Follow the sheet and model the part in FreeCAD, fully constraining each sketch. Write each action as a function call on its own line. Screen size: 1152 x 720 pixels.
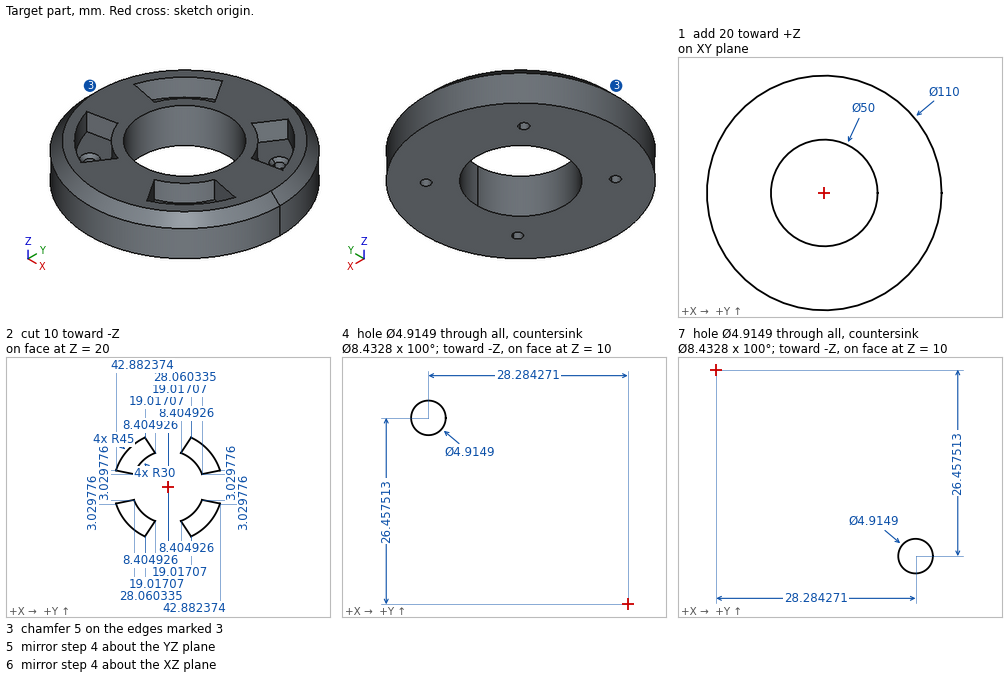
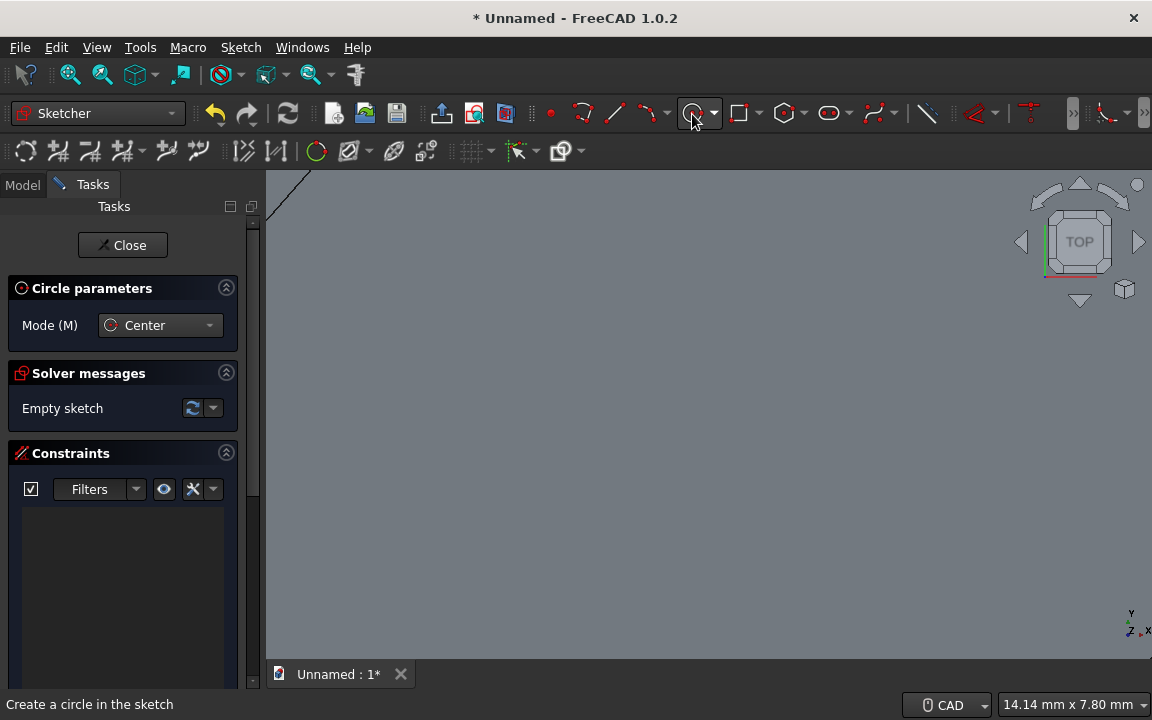
click(625, 402)
click(734, 293)
key(Escape)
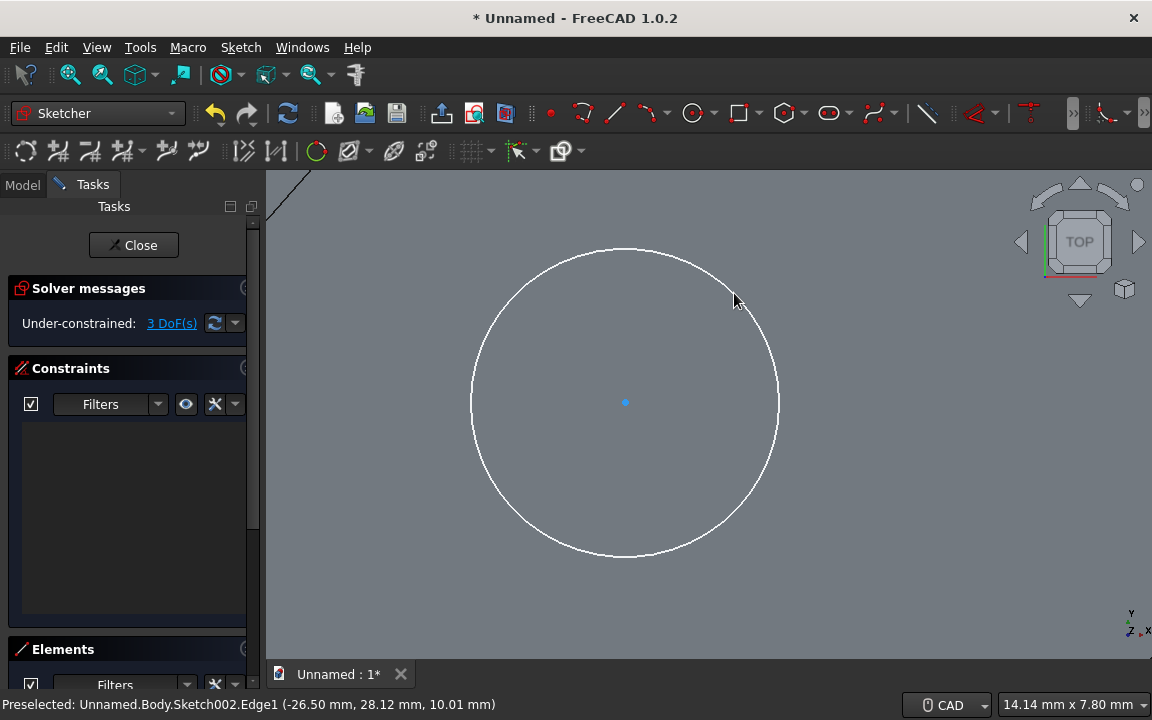
click(974, 114)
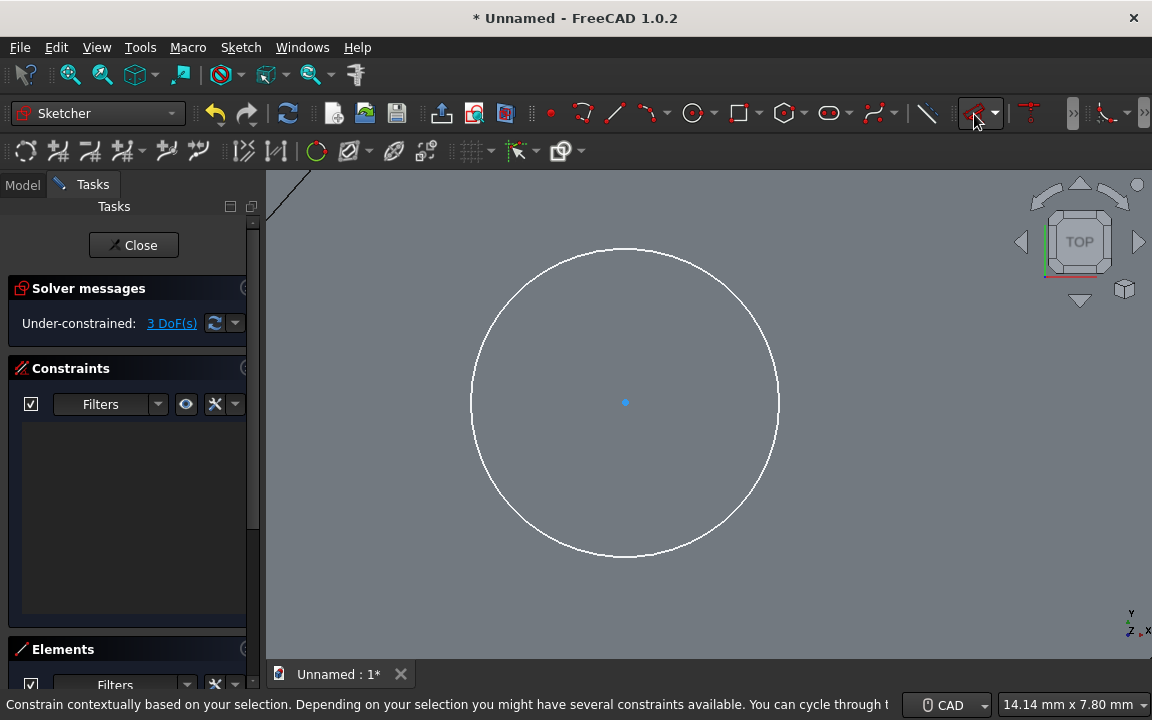
click(734, 294)
click(757, 271)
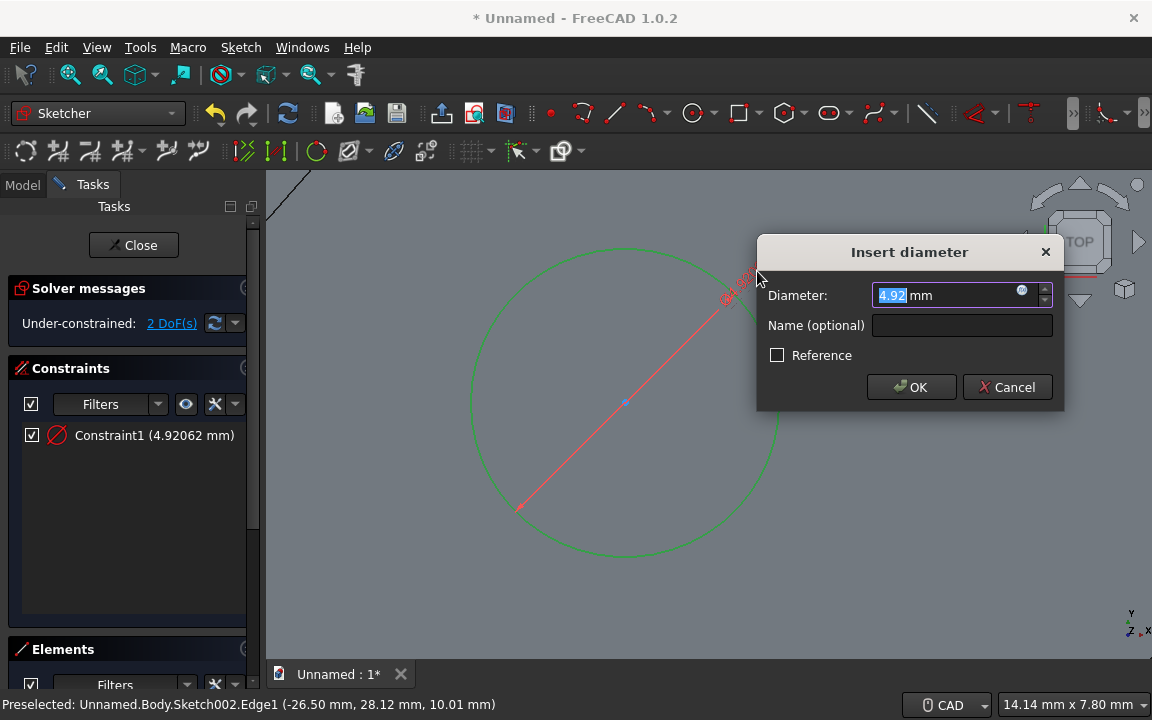
text(4.9149)
key(Return)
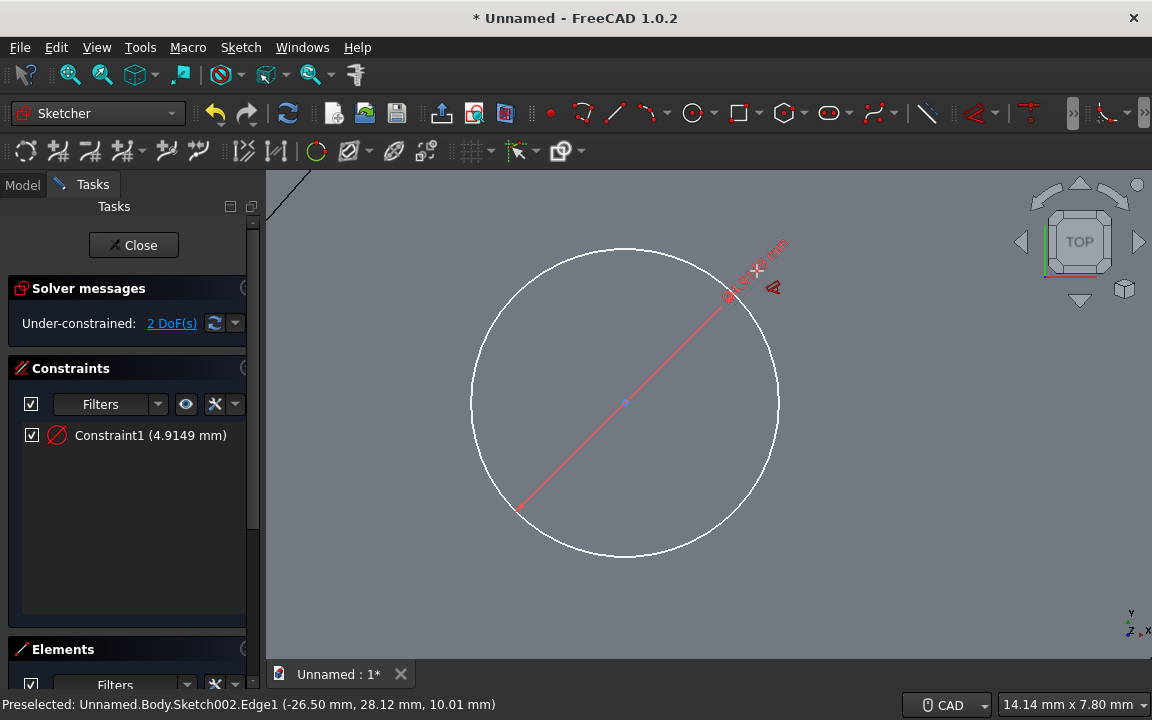
click(625, 403)
click(806, 369)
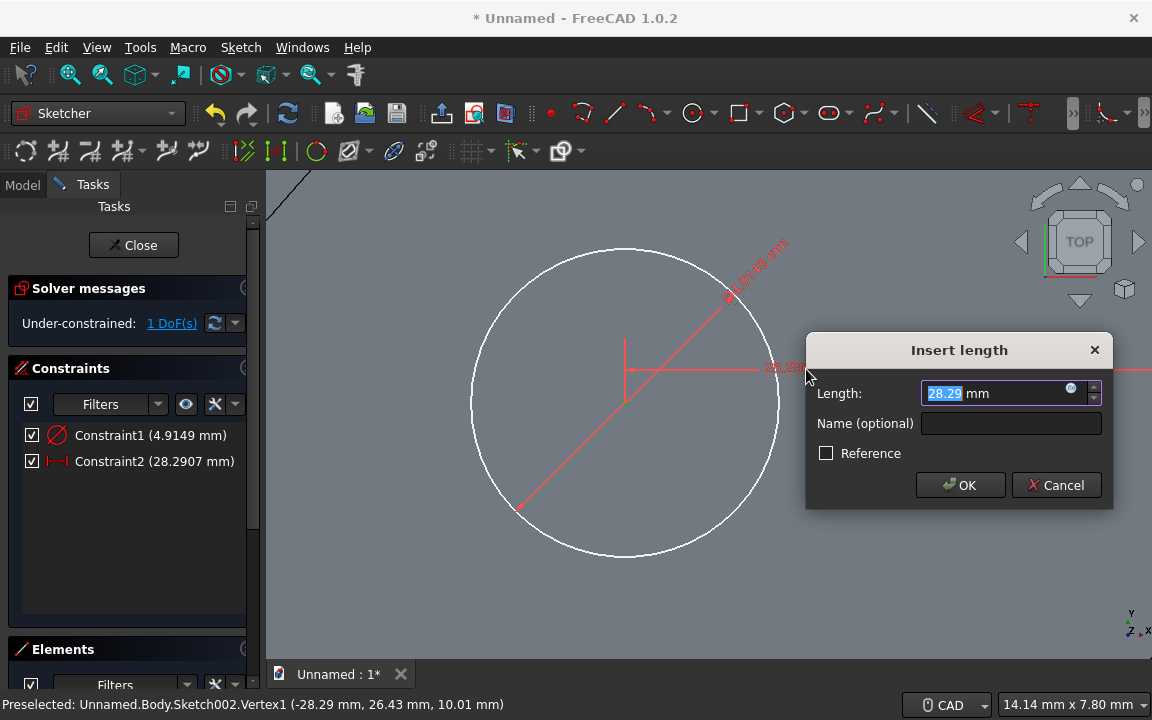
text(28.284271)
key(Return)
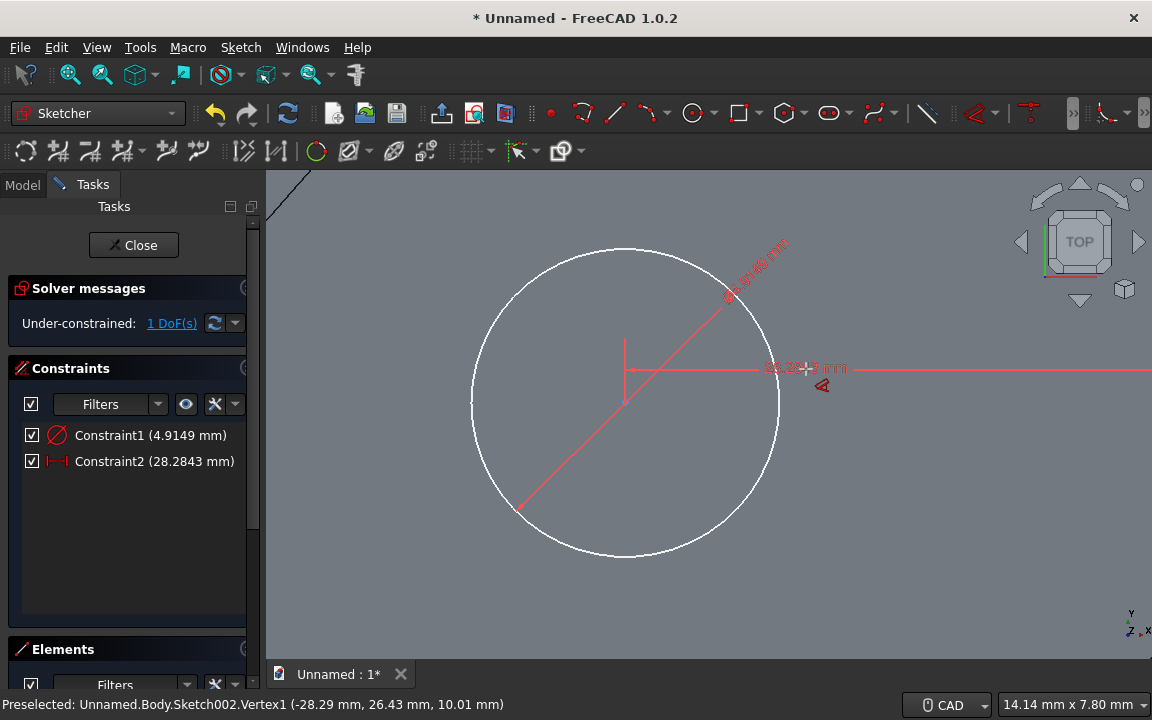
click(625, 403)
click(591, 517)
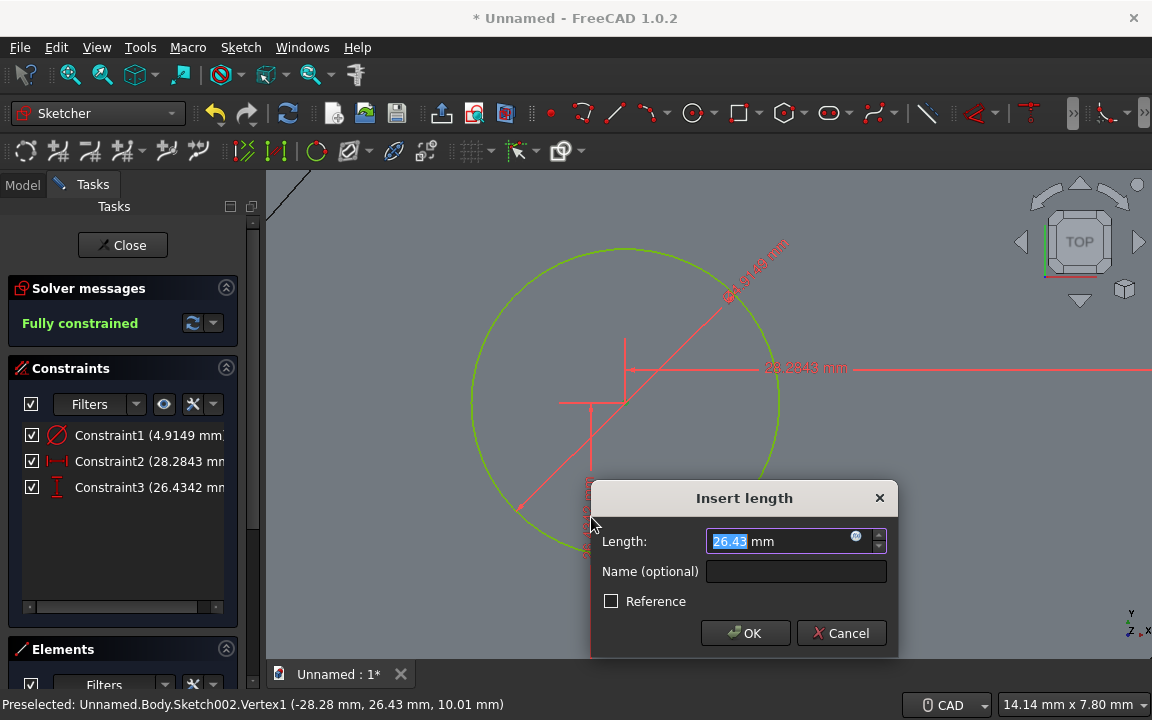
text(26.457513)
key(Return)
key(Escape)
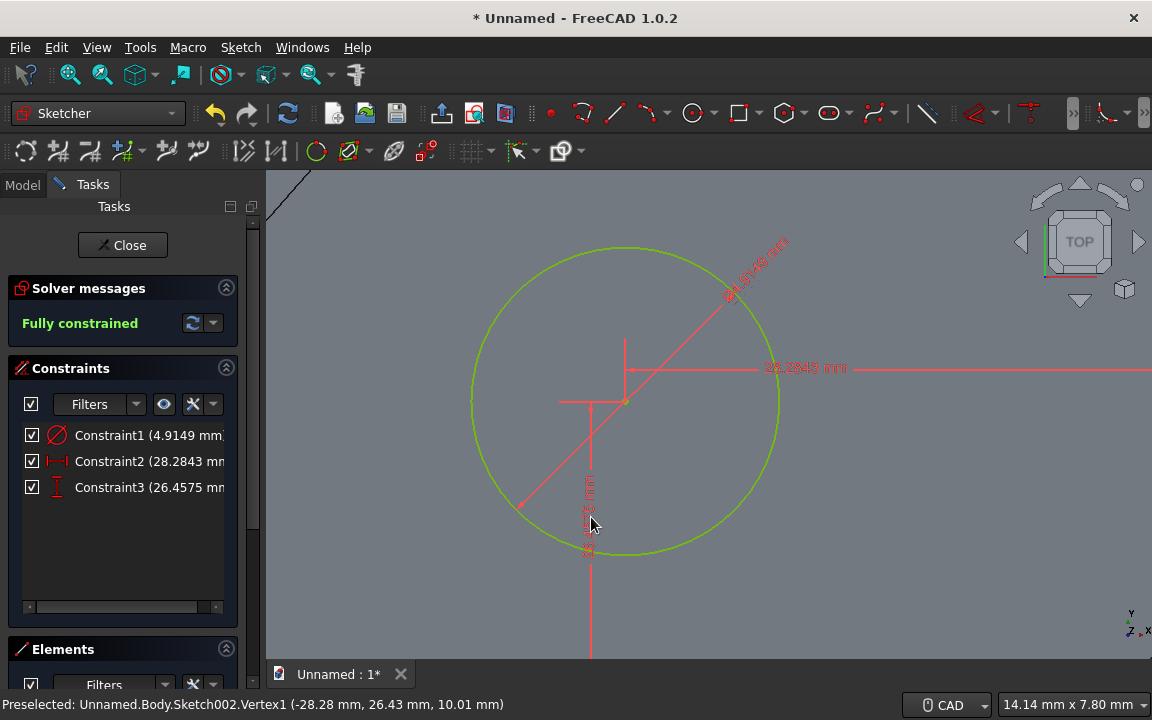
click(123, 245)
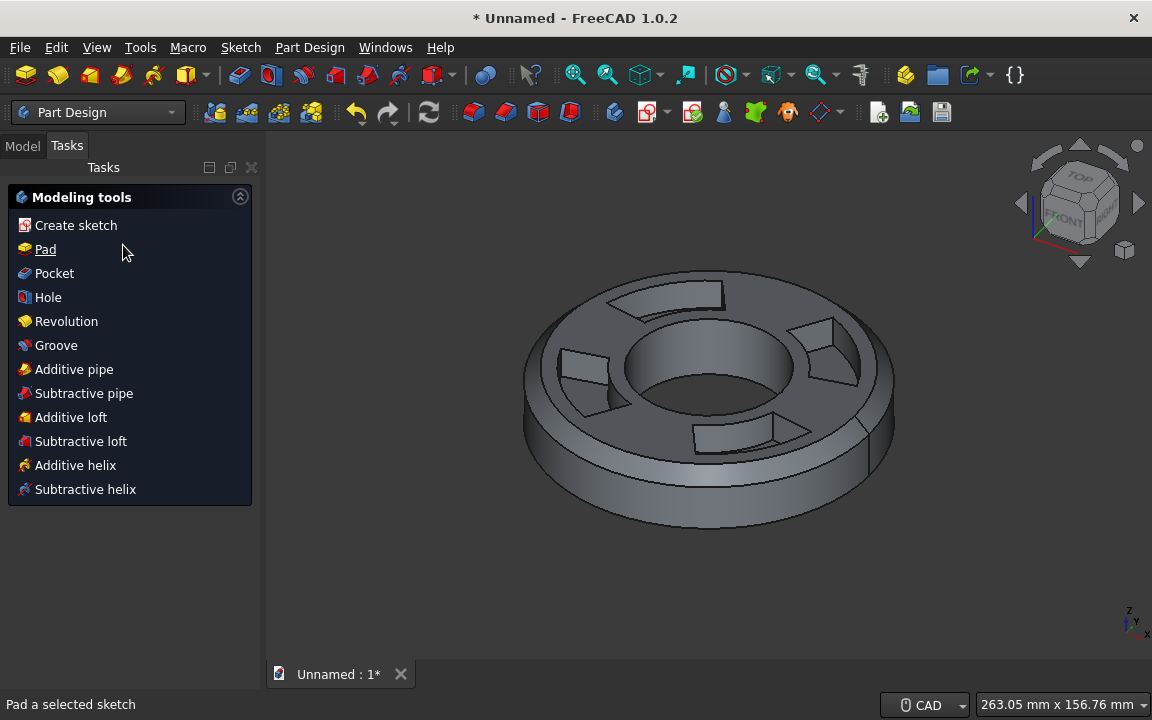
click(272, 76)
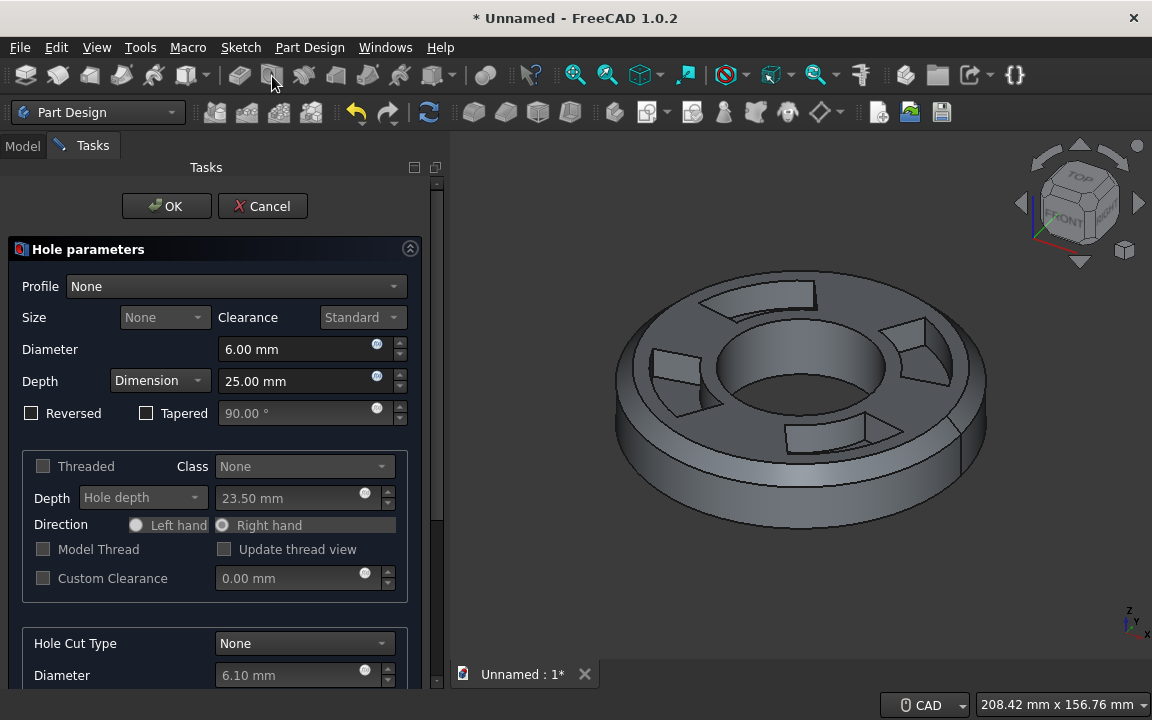
triple_click(305, 349)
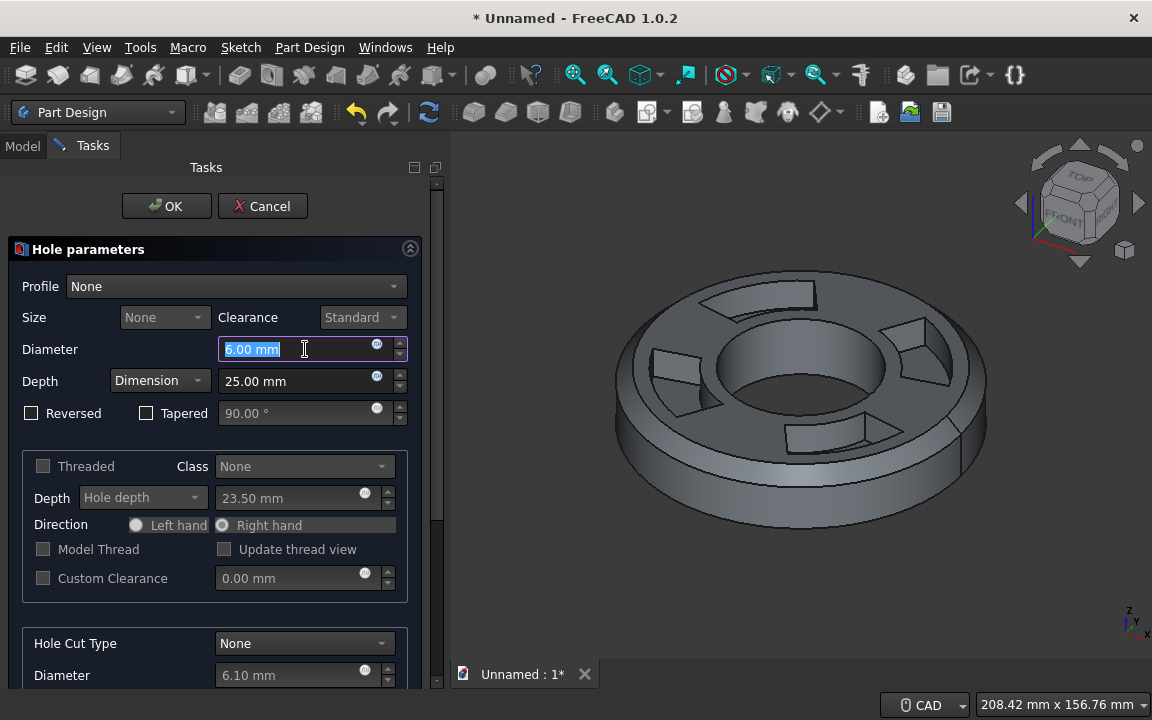
text(4.9149)
key(Tab)